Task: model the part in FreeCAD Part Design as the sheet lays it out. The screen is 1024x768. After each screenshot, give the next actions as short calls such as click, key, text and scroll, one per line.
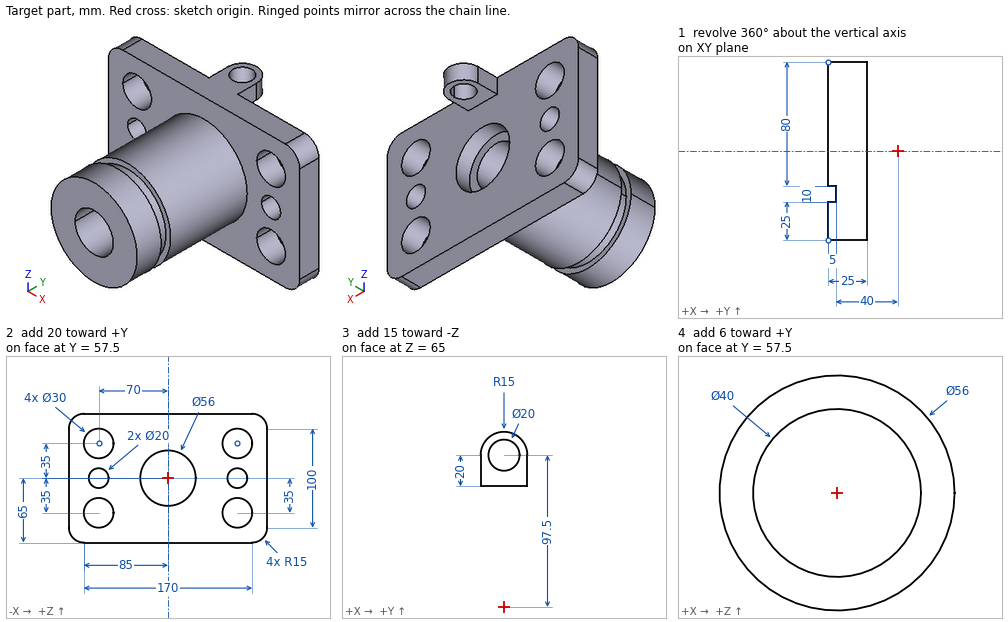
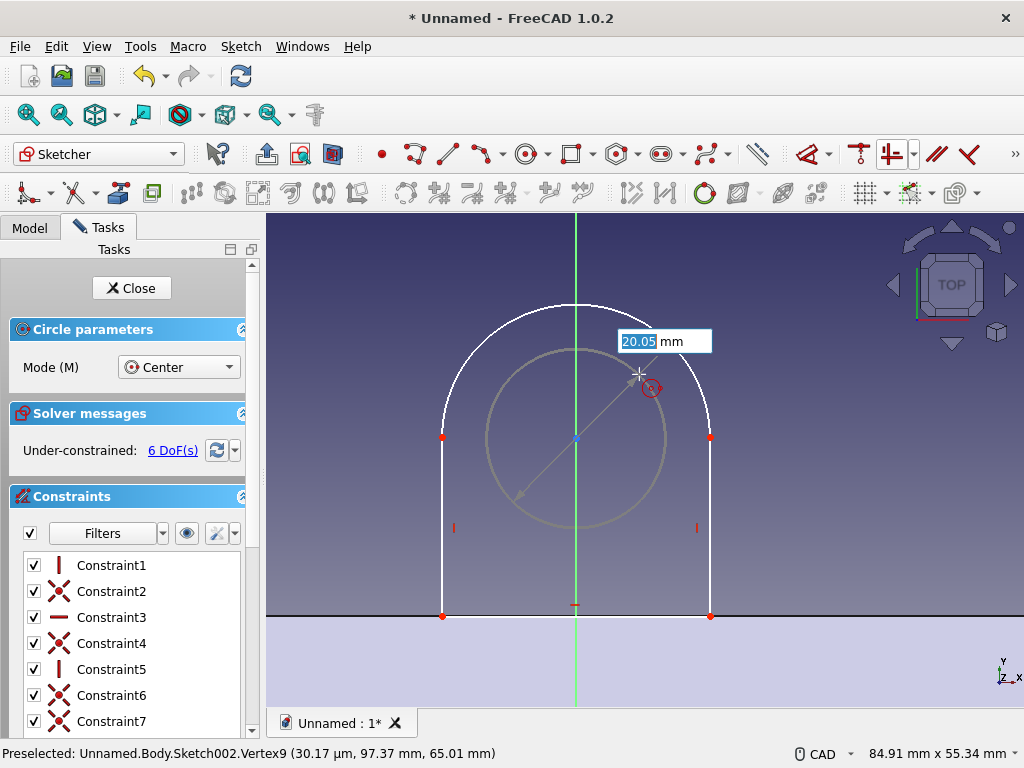
text(20)
key(Return)
key(Escape)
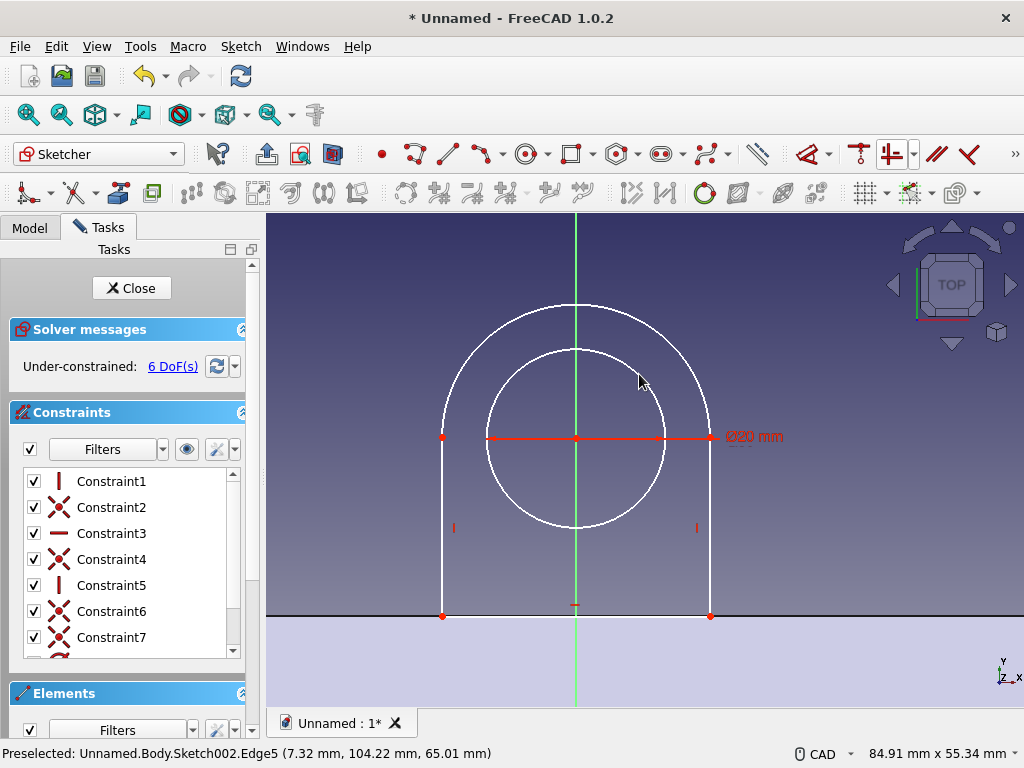
click(442, 492)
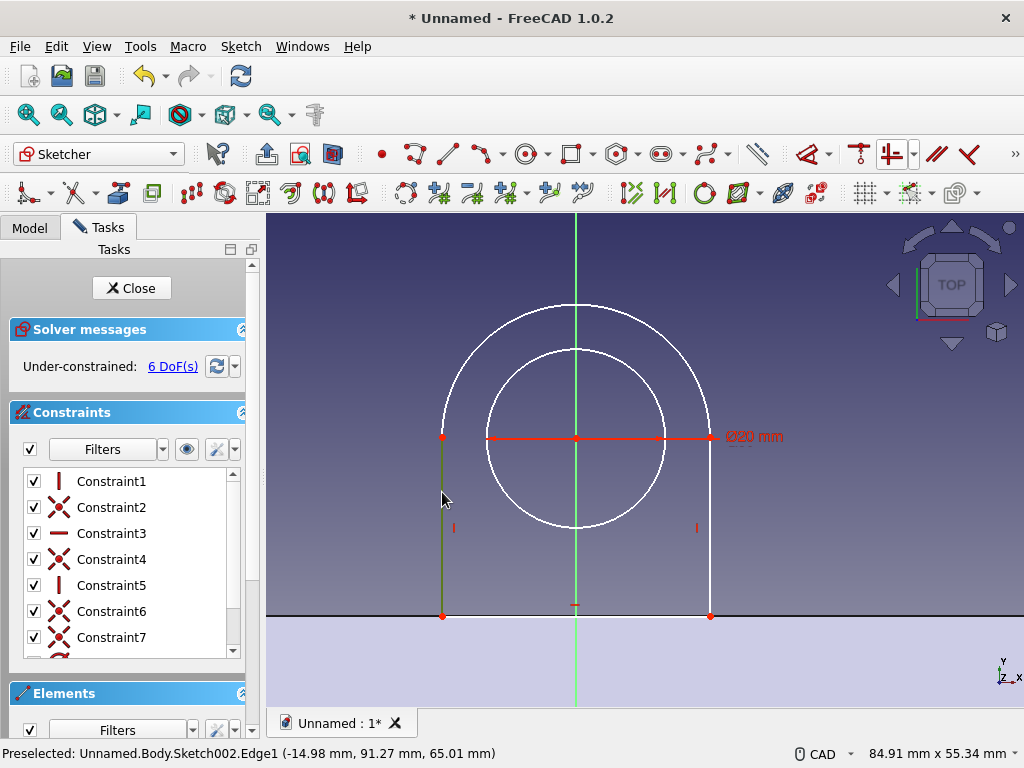
click(655, 330)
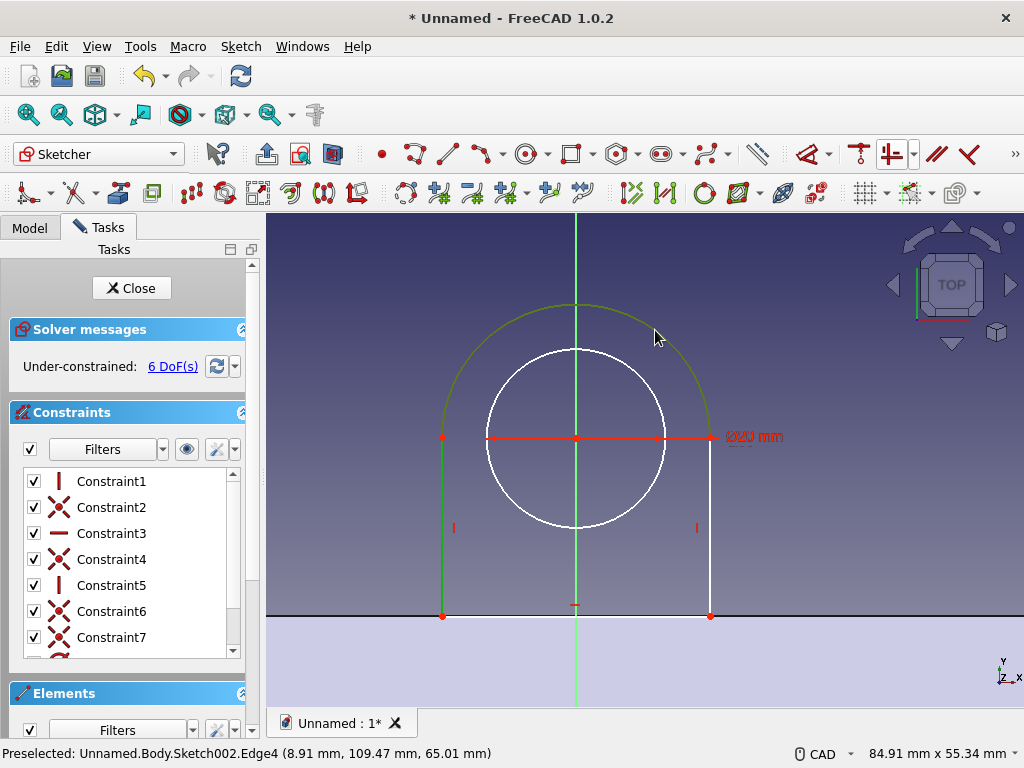
key(t)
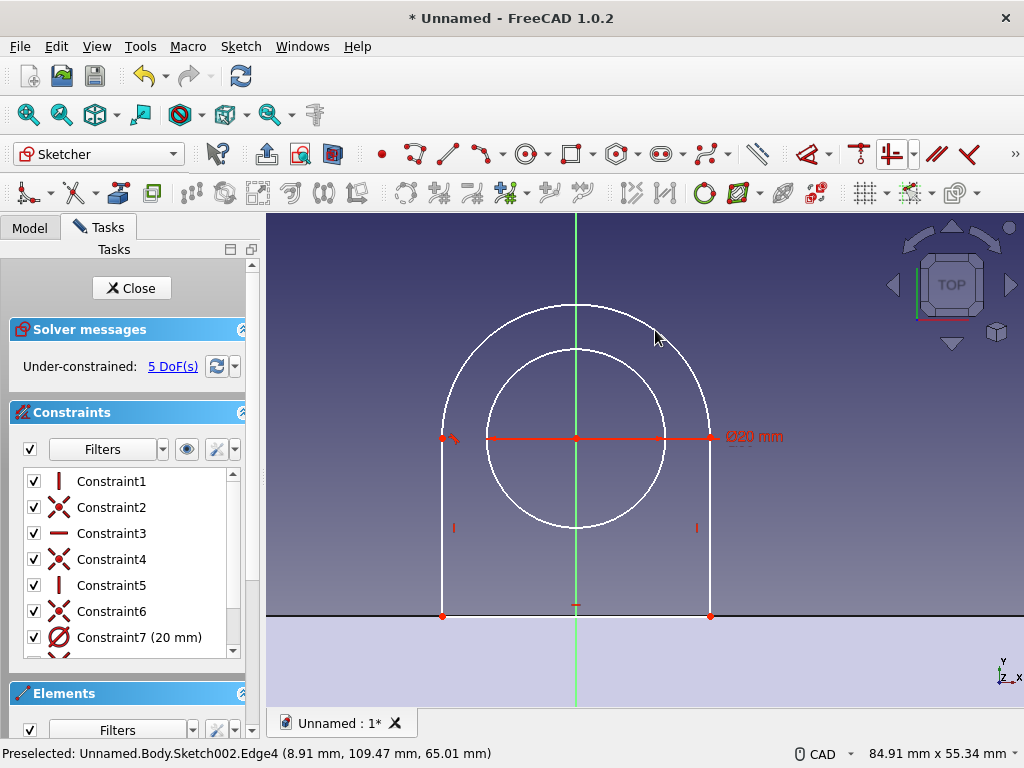
click(710, 563)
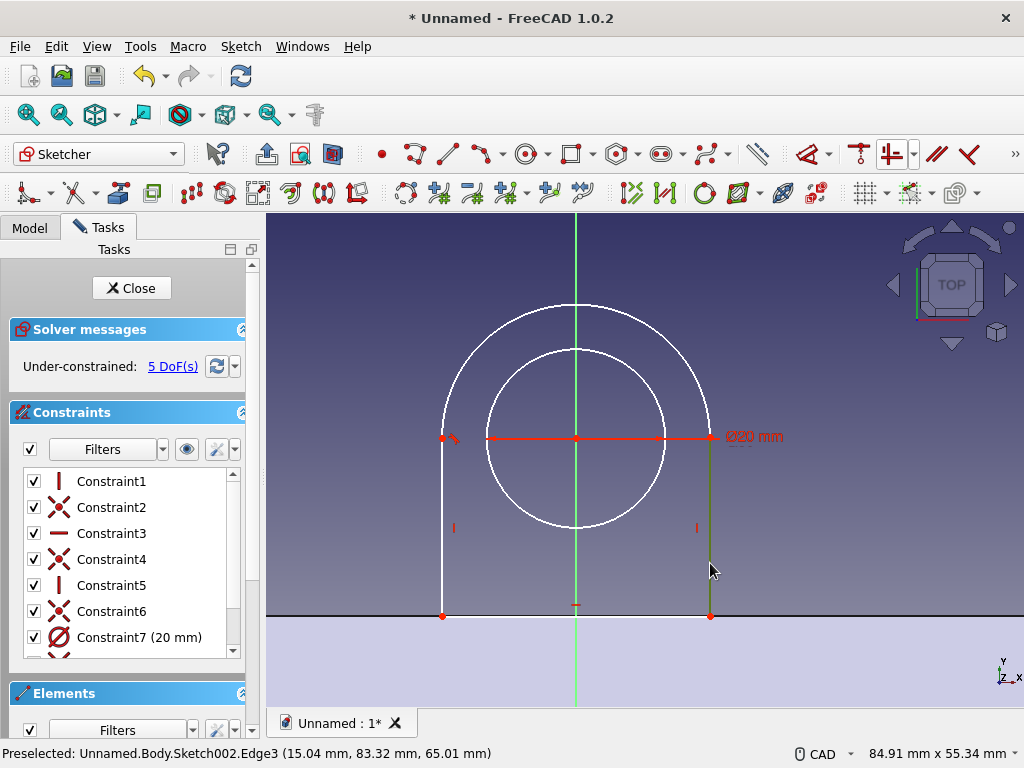
click(654, 330)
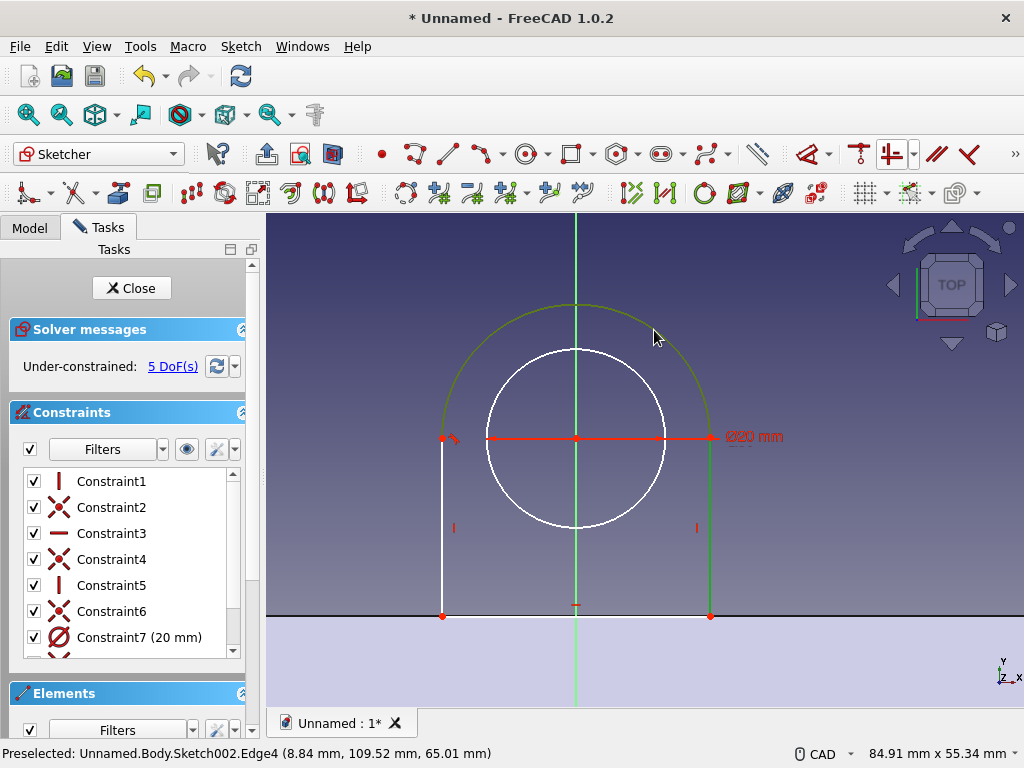
key(t)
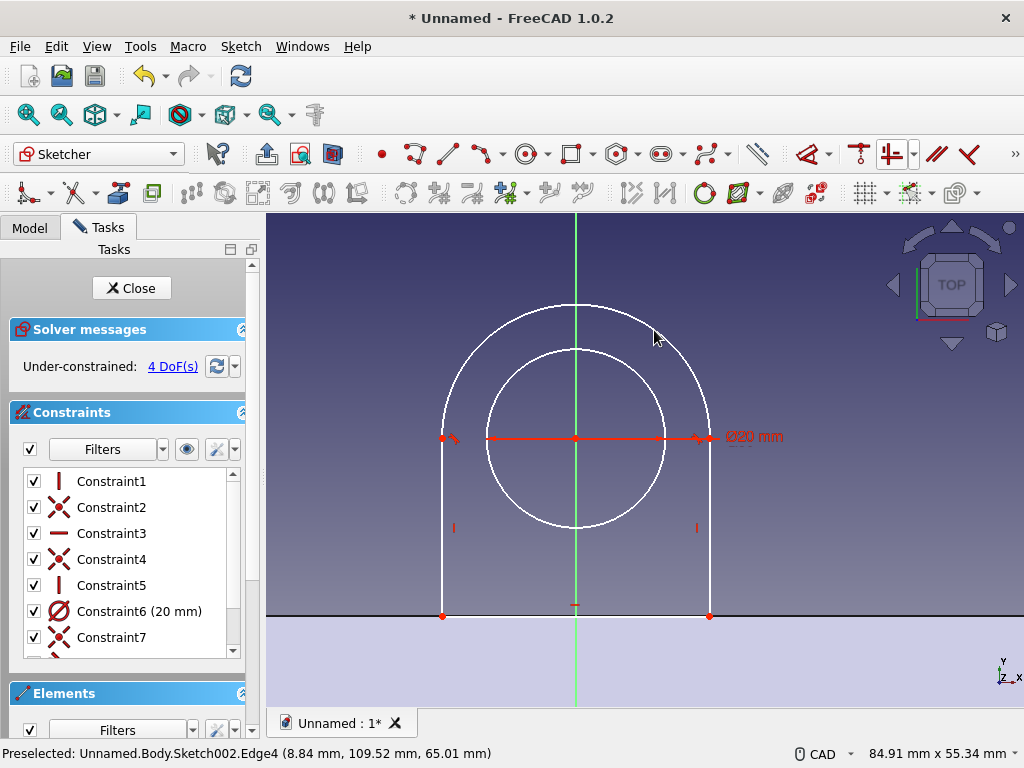
click(576, 439)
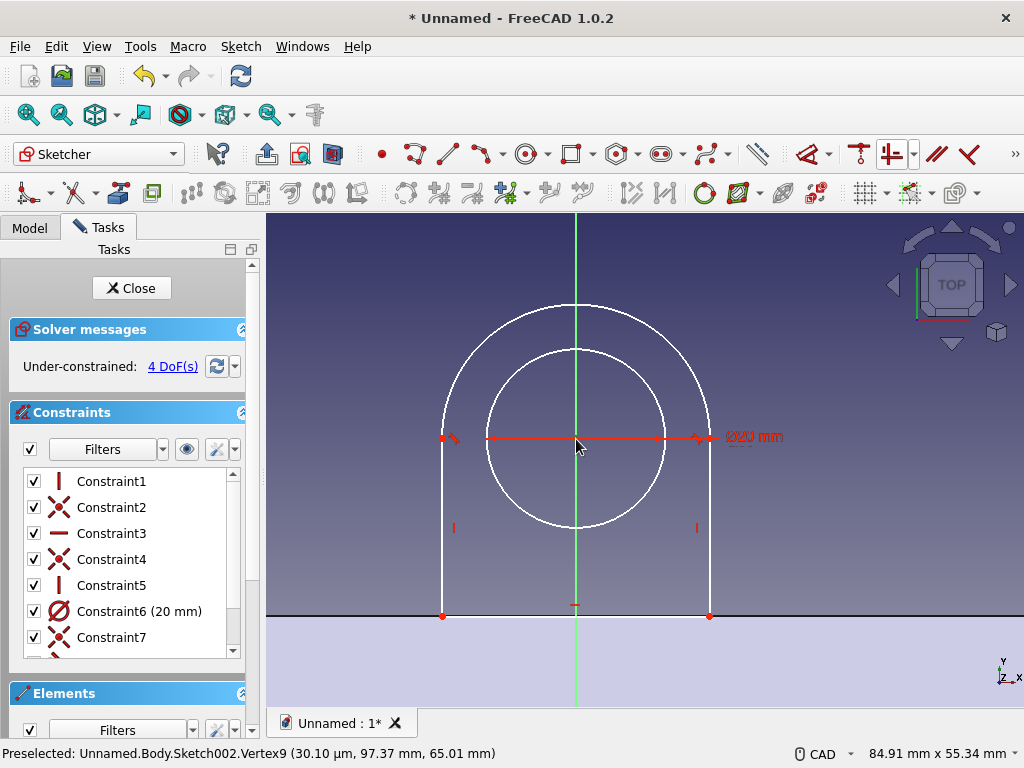
click(576, 648)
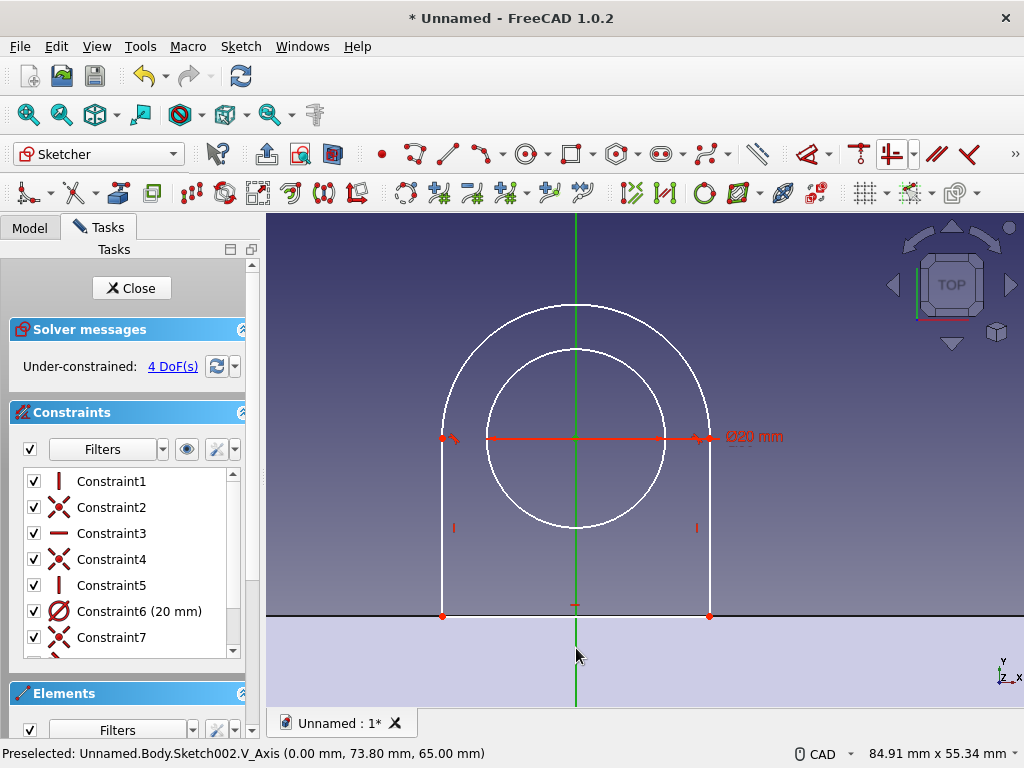
click(859, 154)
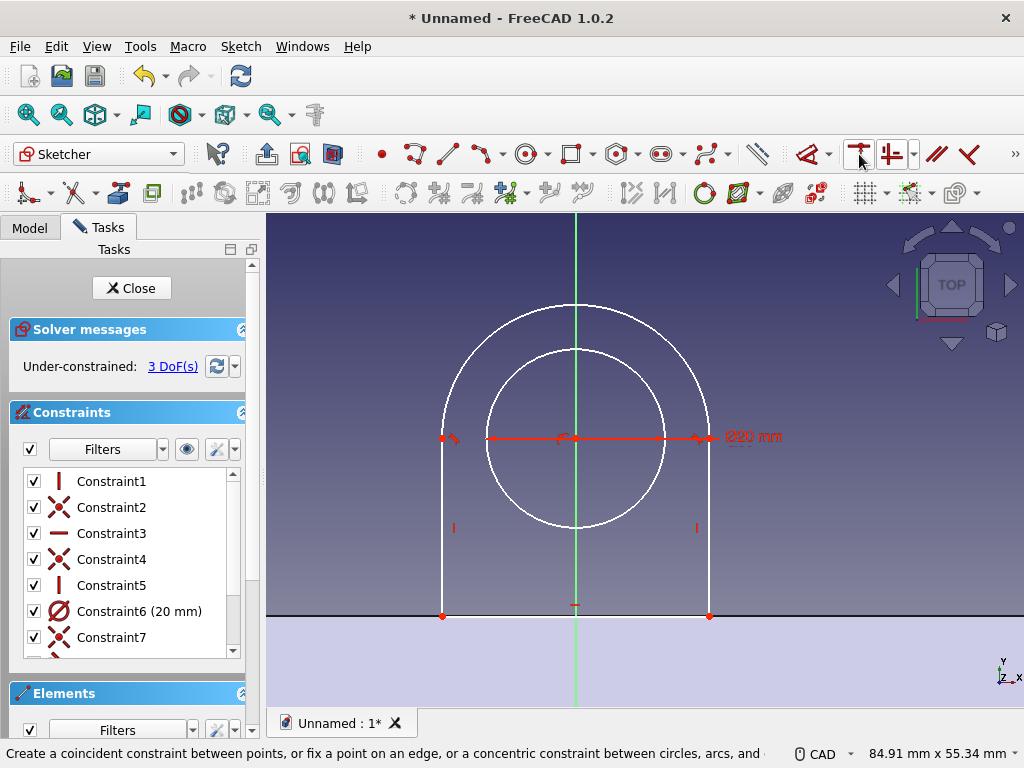
click(806, 154)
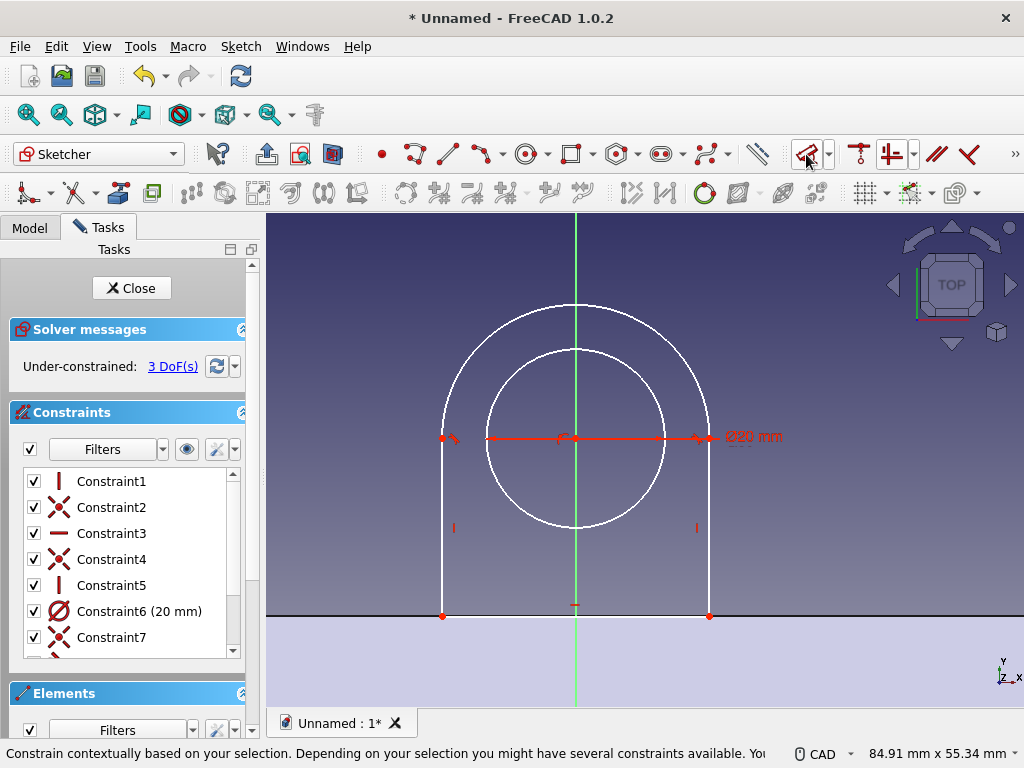
click(654, 330)
click(673, 304)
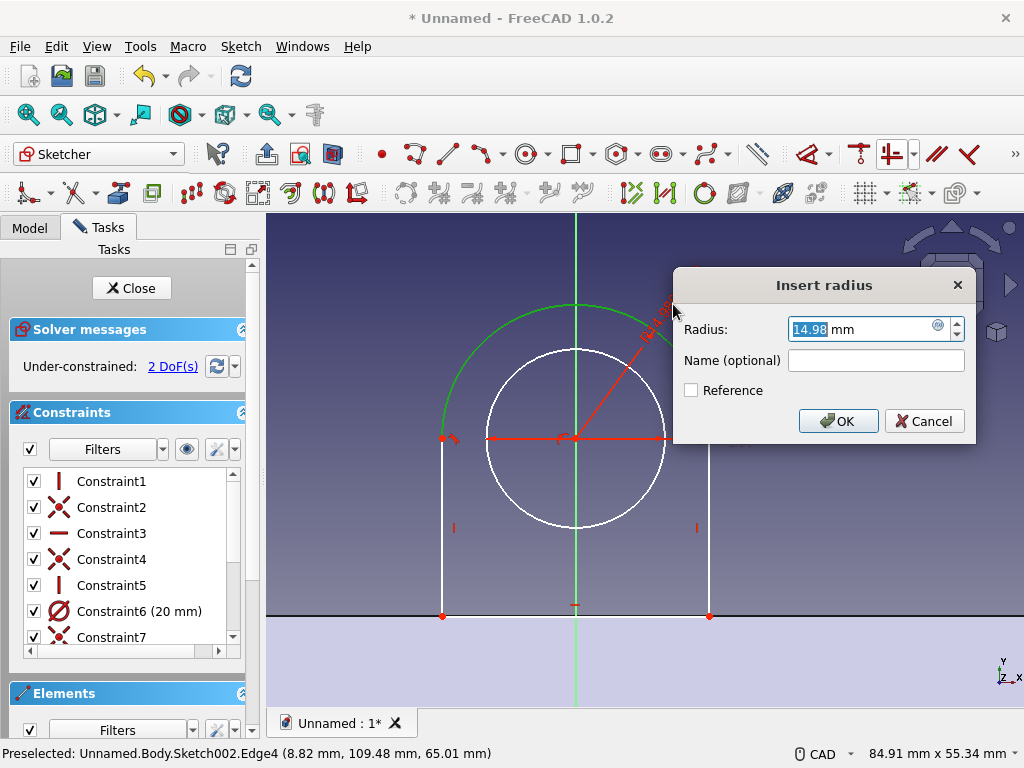
text(15)
key(Return)